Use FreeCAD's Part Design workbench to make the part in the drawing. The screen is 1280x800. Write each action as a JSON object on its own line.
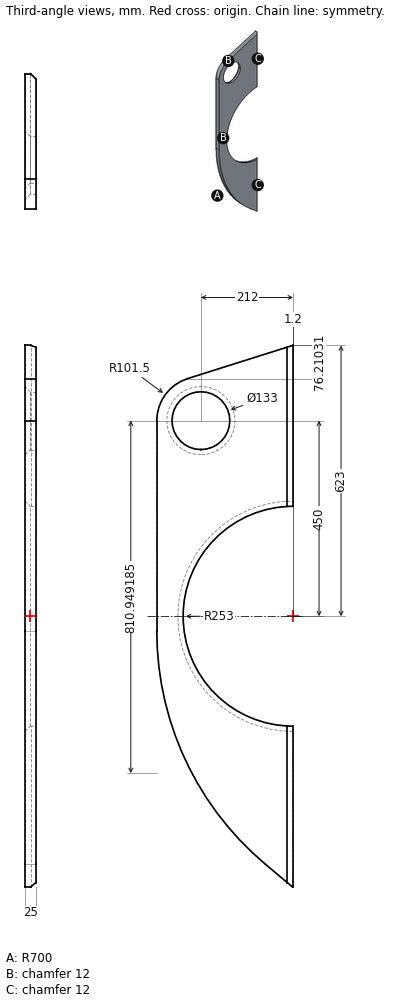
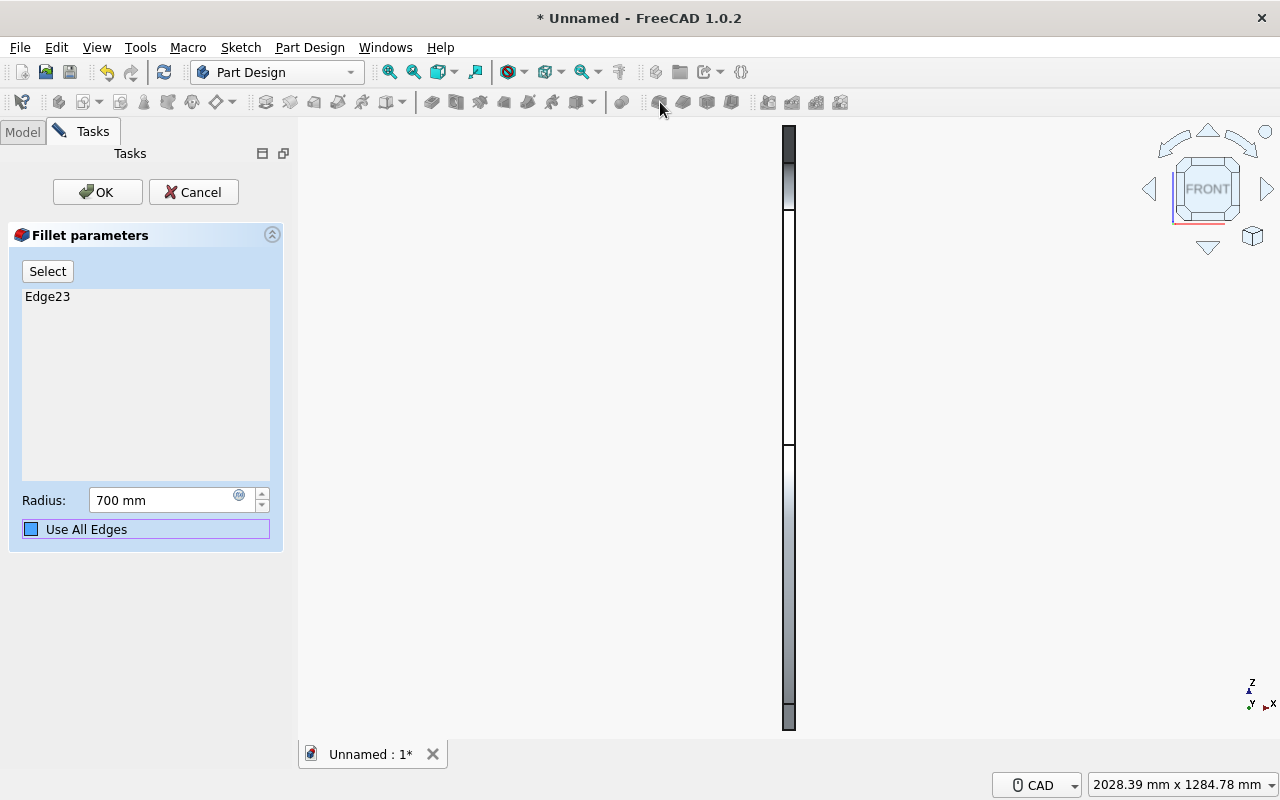
{"action": "left_click", "coordinate": [98, 192]}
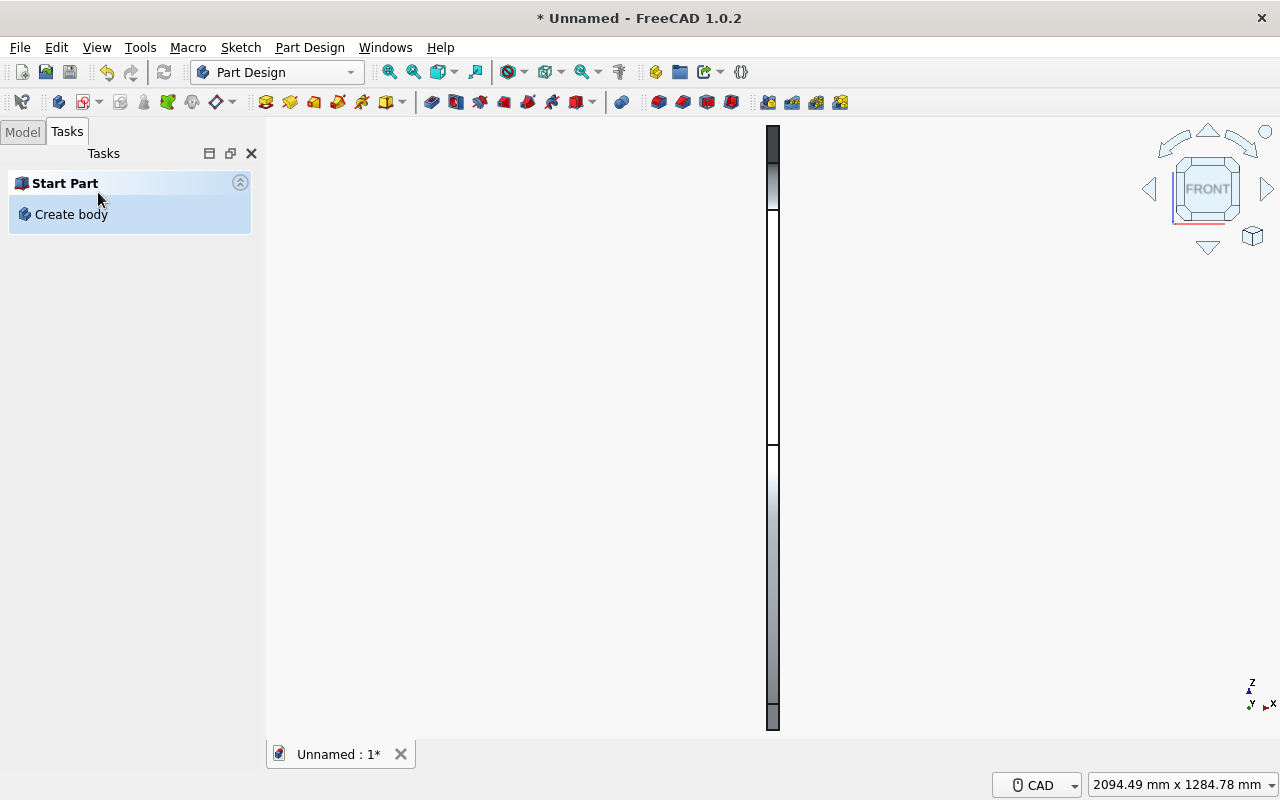
{"action": "key", "text": "0"}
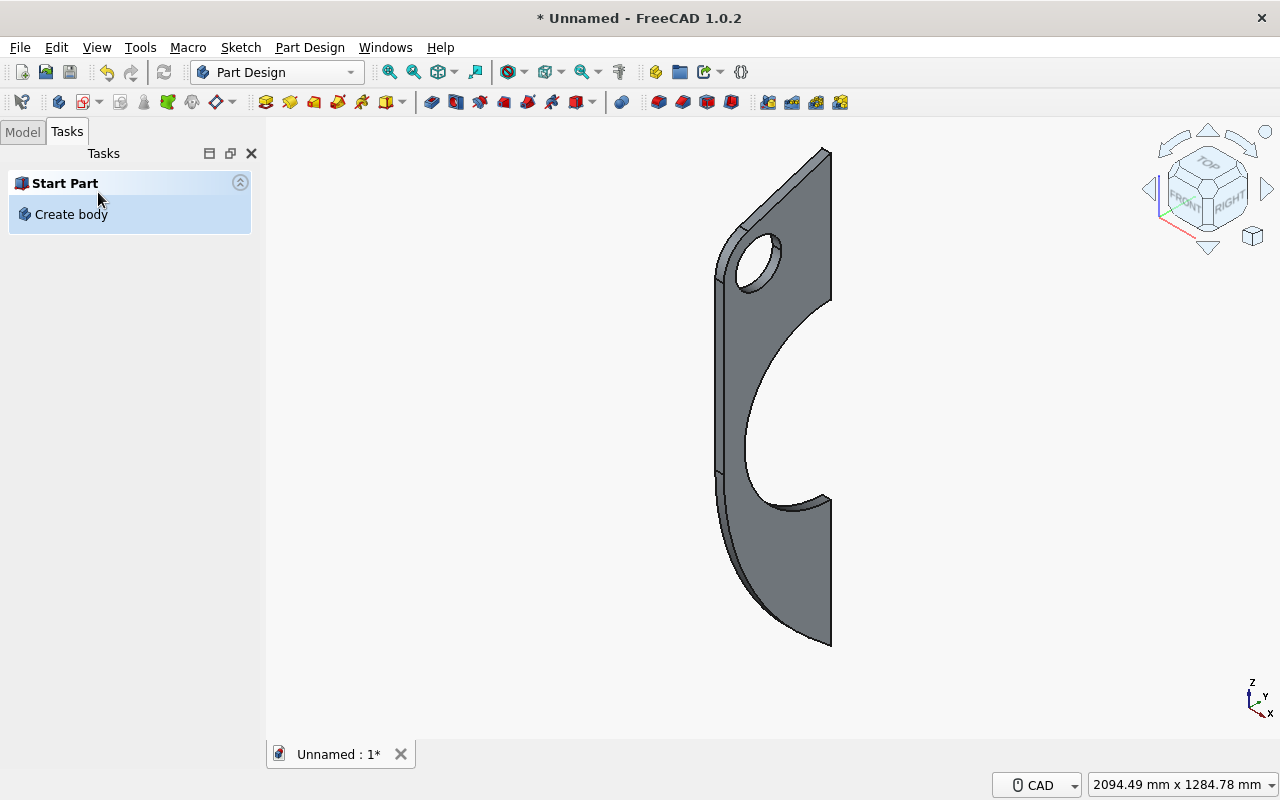
{"action": "key", "text": "2"}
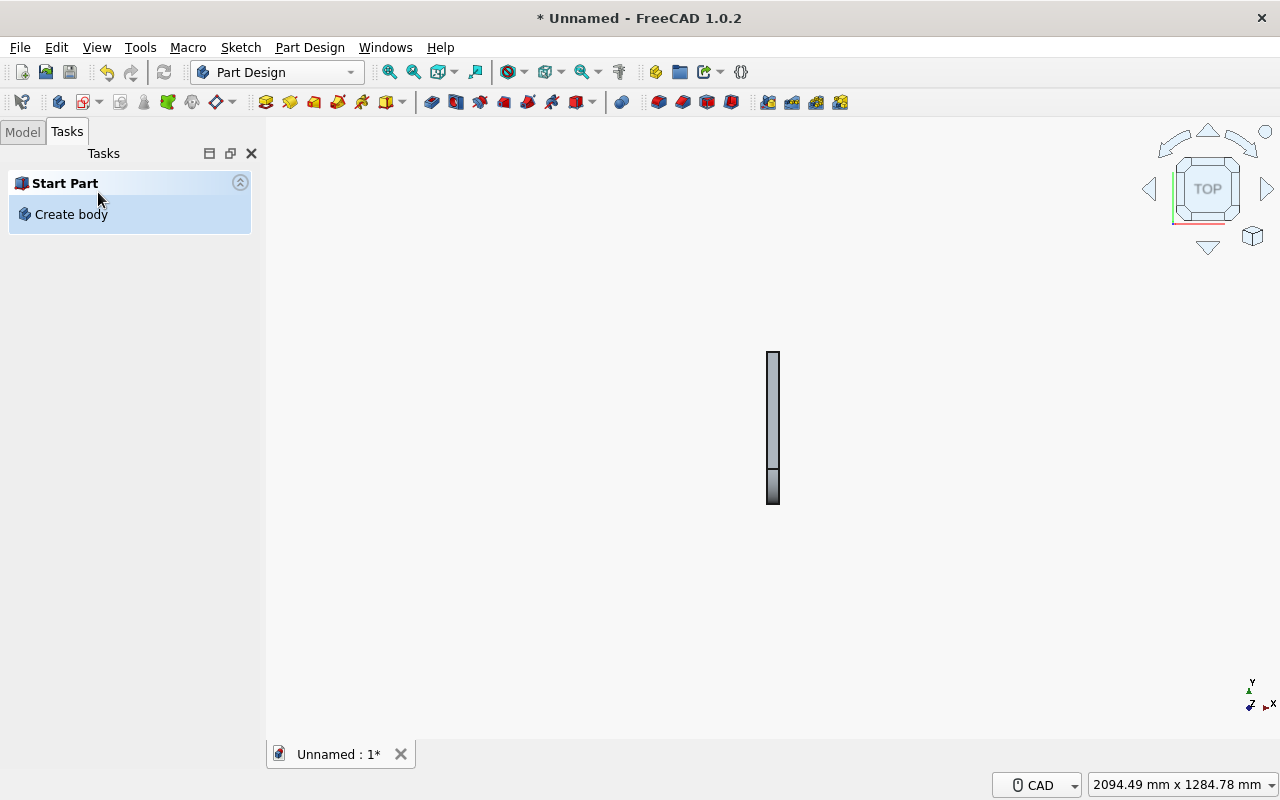
{"action": "left_click", "coordinate": [390, 72]}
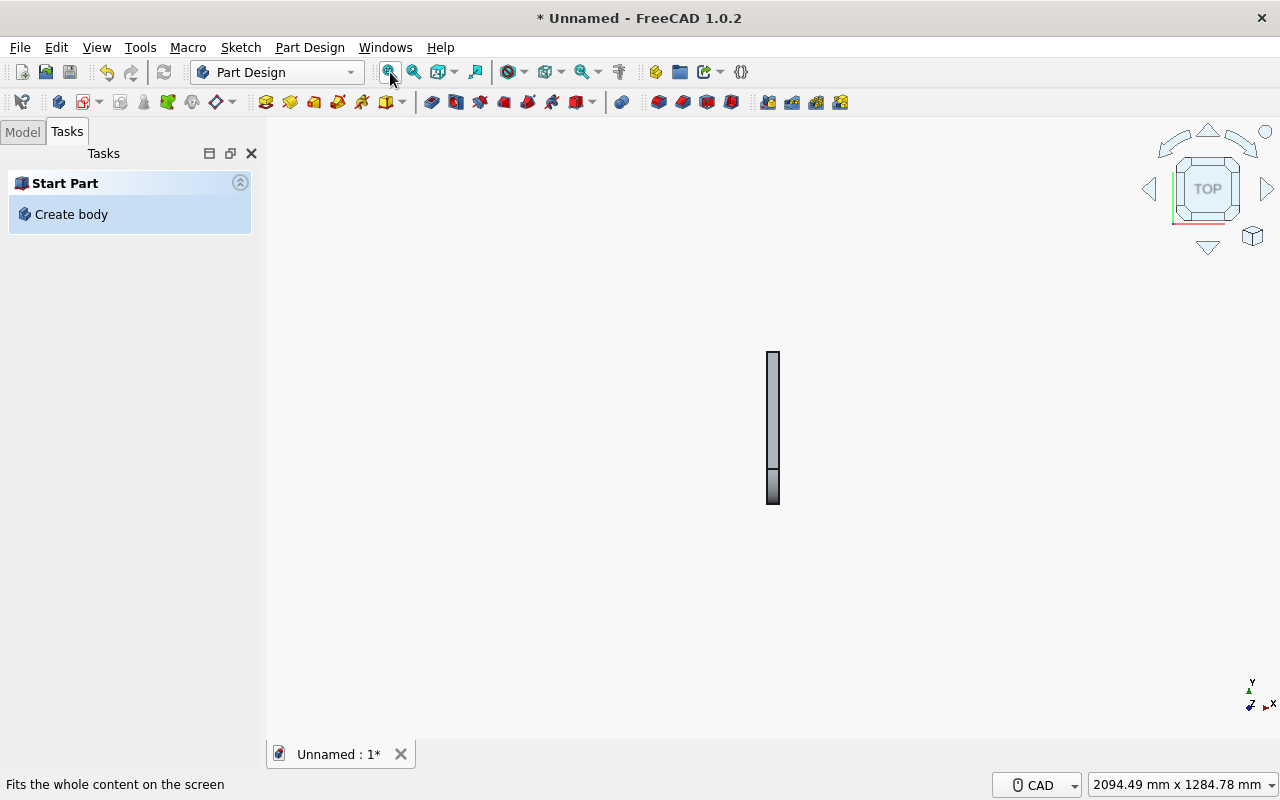
{"action": "key", "text": "1"}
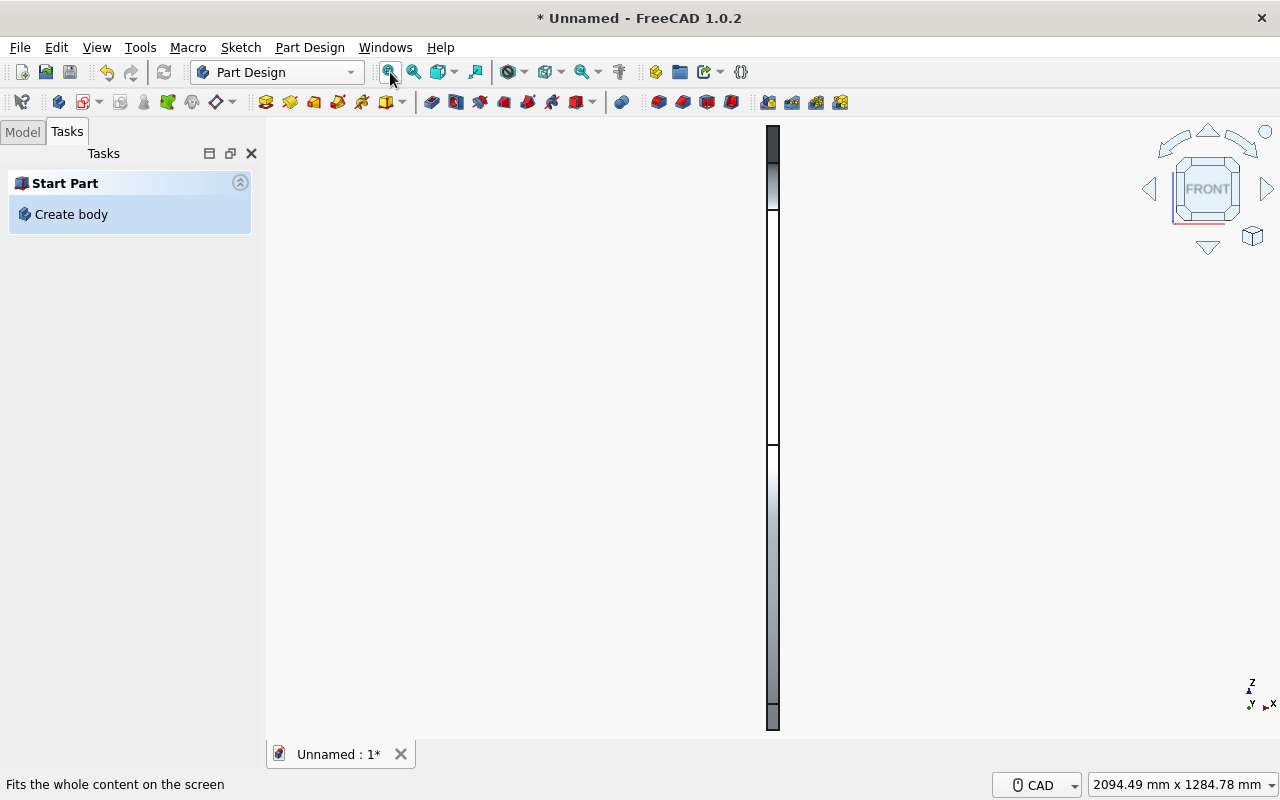
{"action": "key", "text": "3"}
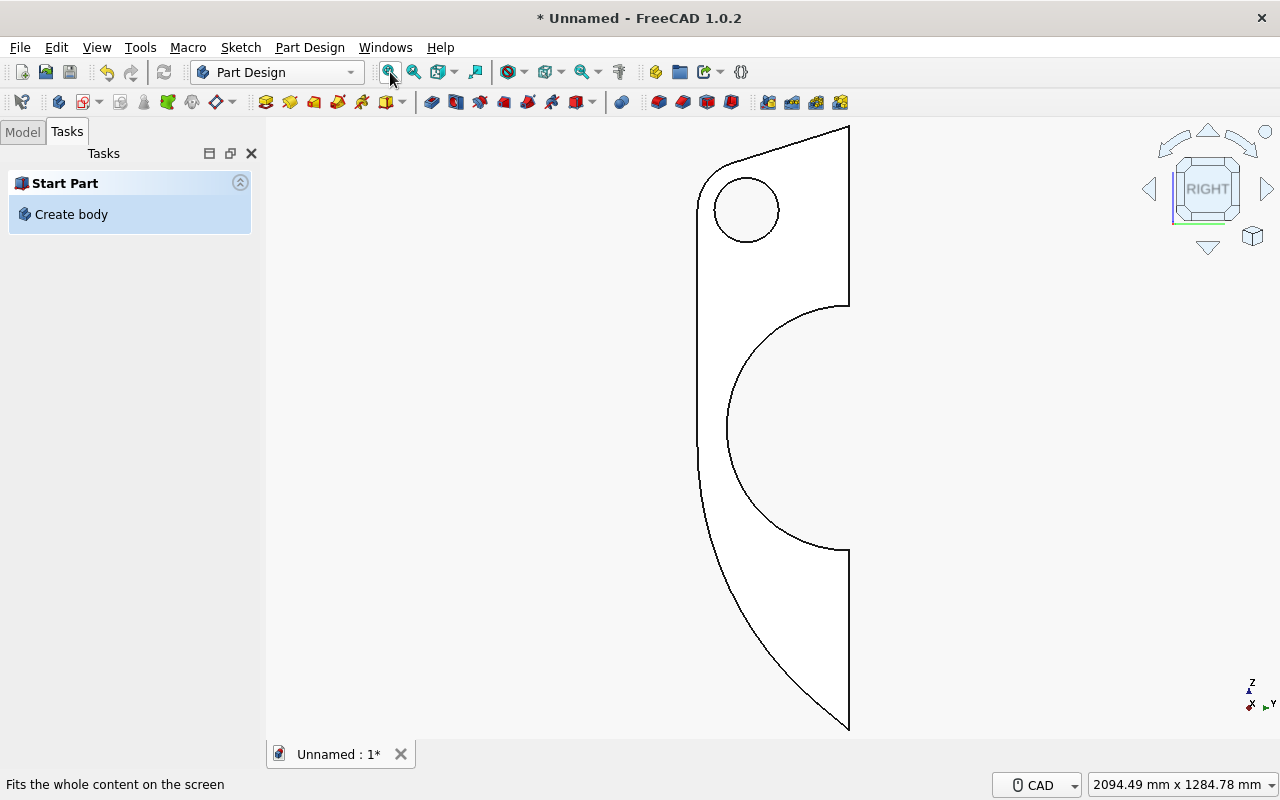
{"action": "key", "text": "5"}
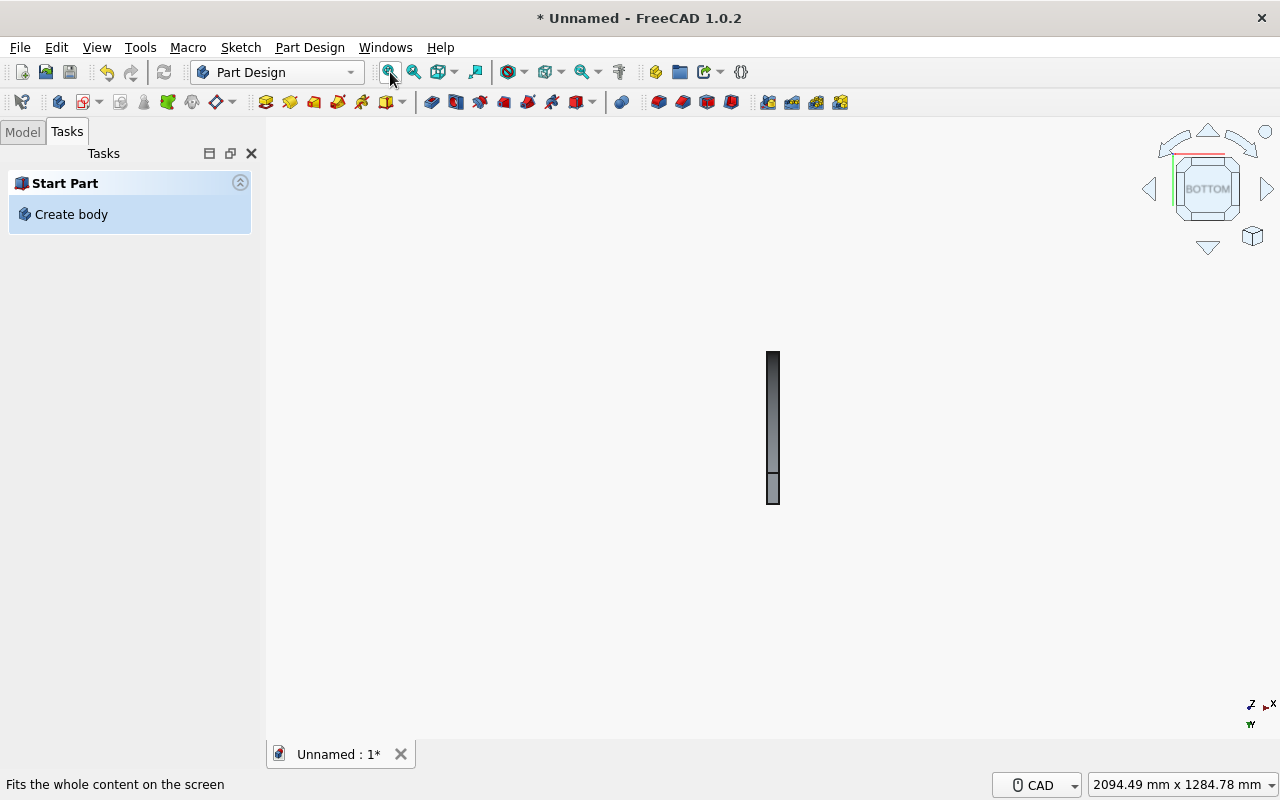
{"action": "left_click", "coordinate": [390, 72]}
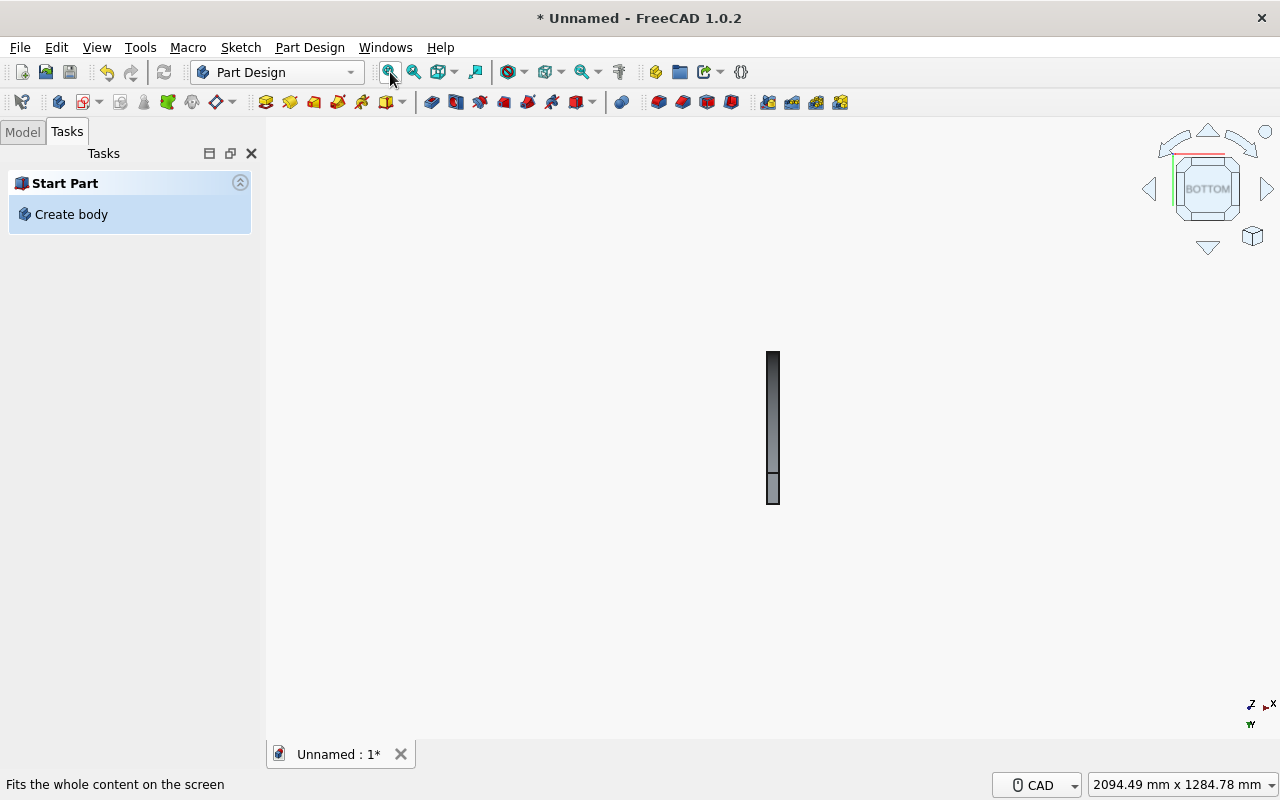
{"action": "key", "text": "4"}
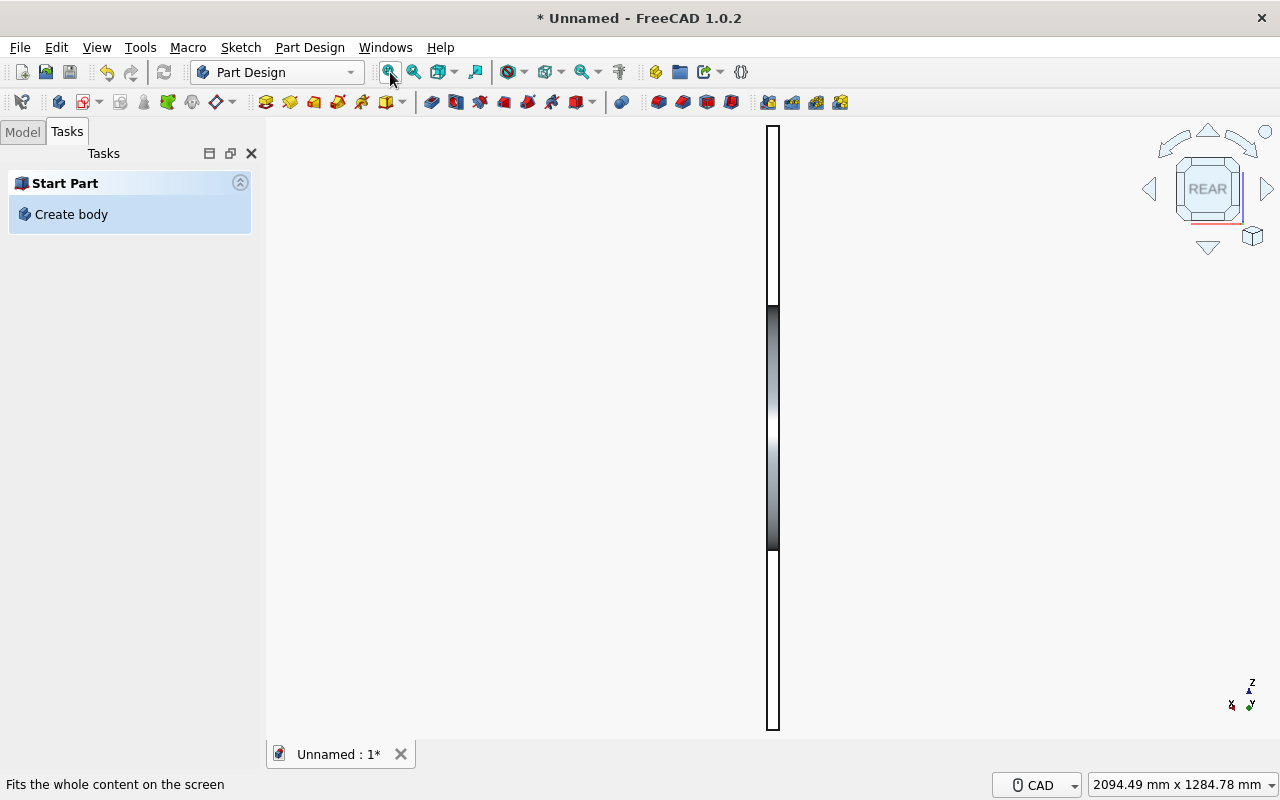
{"action": "left_click", "coordinate": [779, 427]}